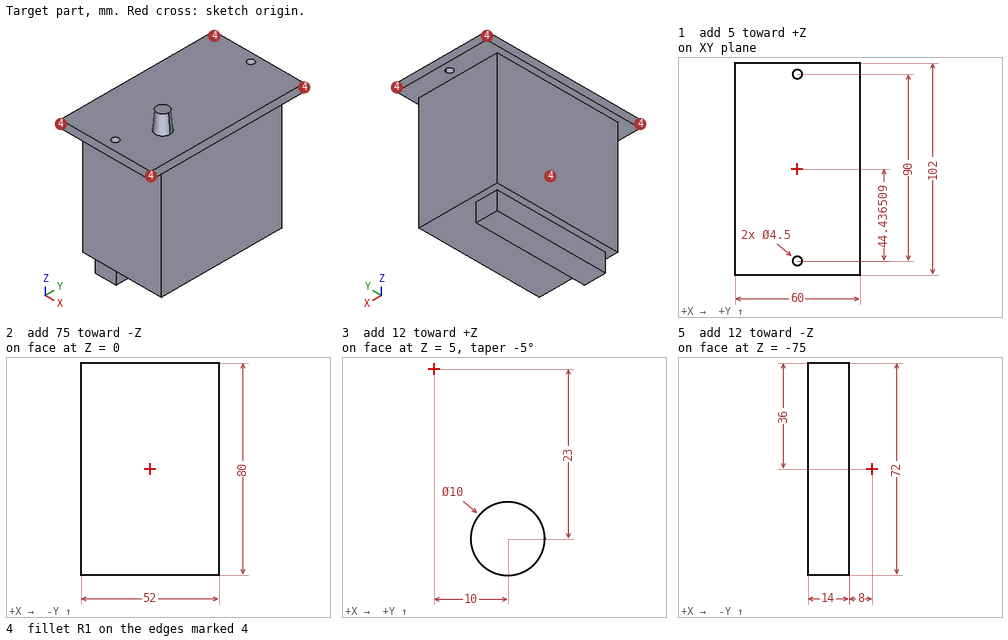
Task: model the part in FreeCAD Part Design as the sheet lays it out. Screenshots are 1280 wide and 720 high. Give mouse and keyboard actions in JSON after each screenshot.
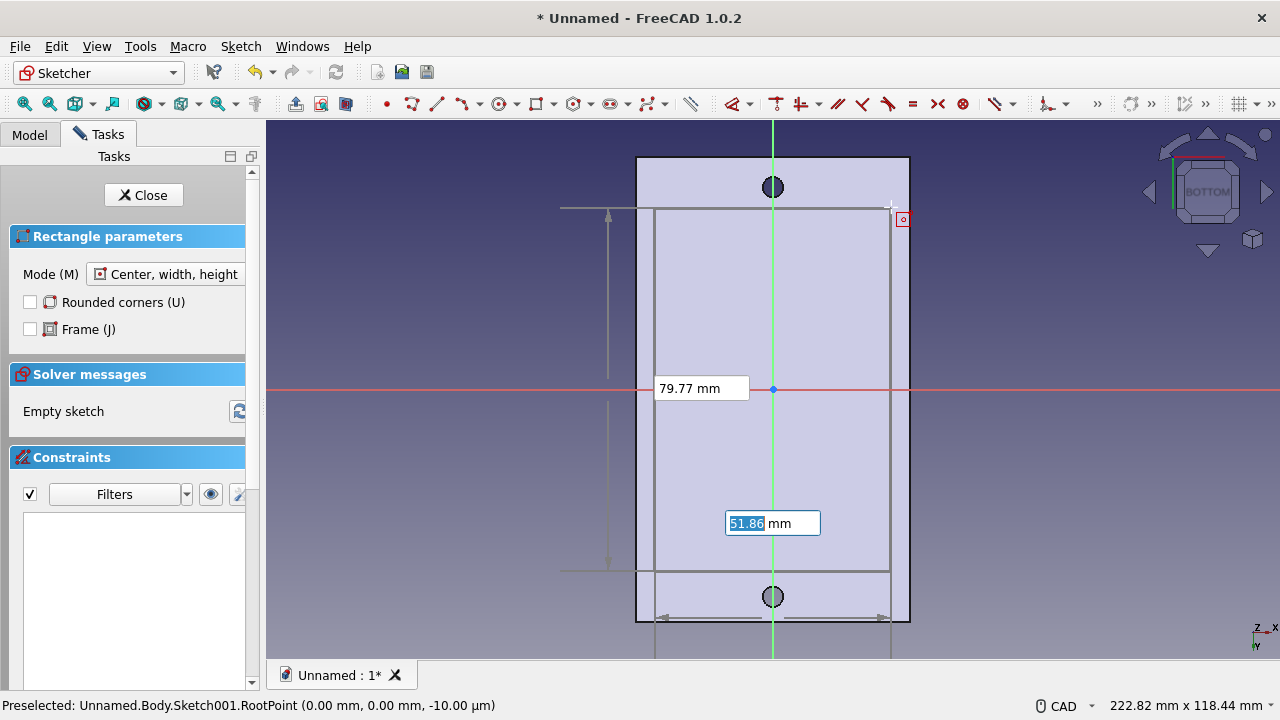
{"action": "type", "text": "52"}
{"action": "key", "text": "Tab"}
{"action": "type", "text": "80"}
{"action": "key", "text": "Return"}
{"action": "key", "text": "Escape"}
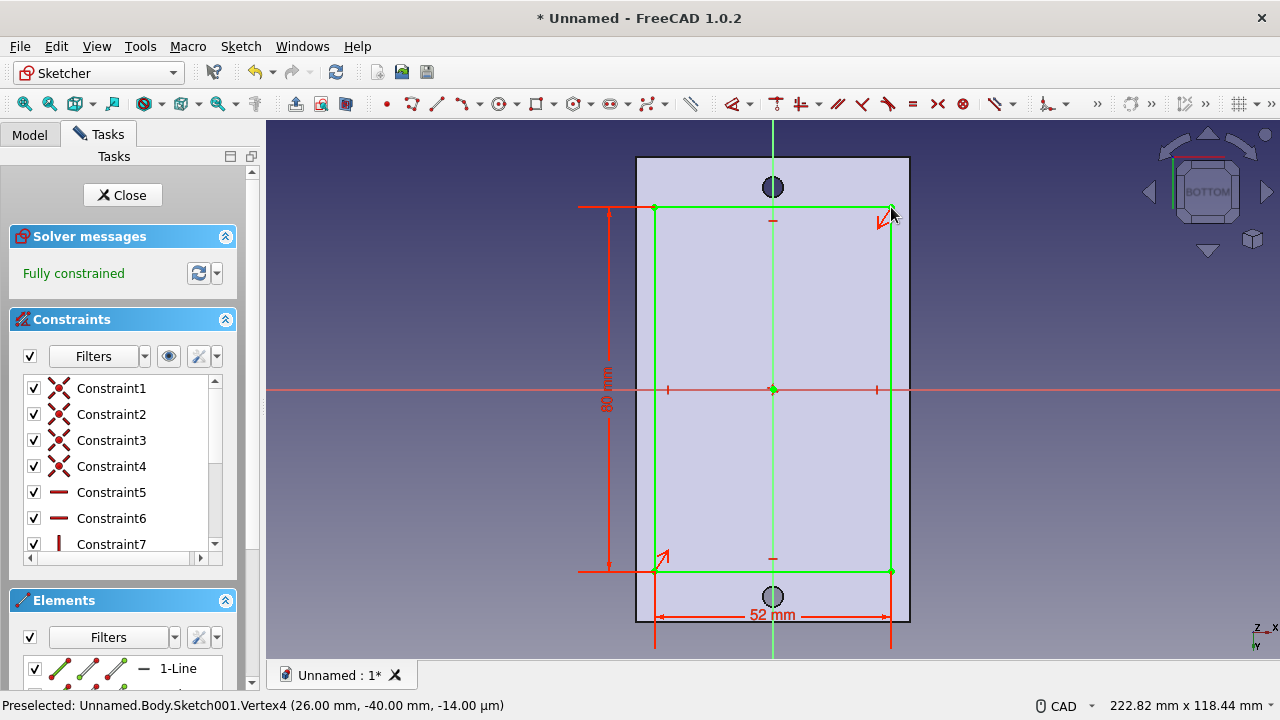
{"action": "left_click", "coordinate": [123, 195]}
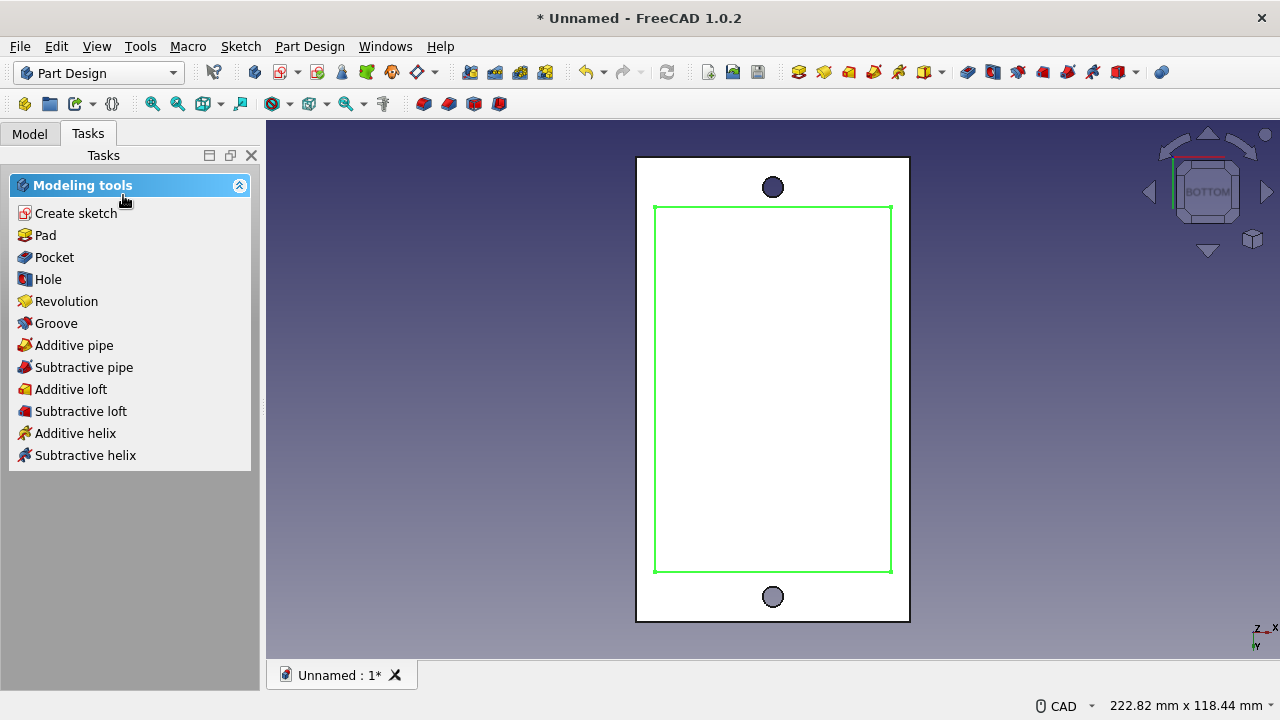
{"action": "left_click", "coordinate": [799, 72]}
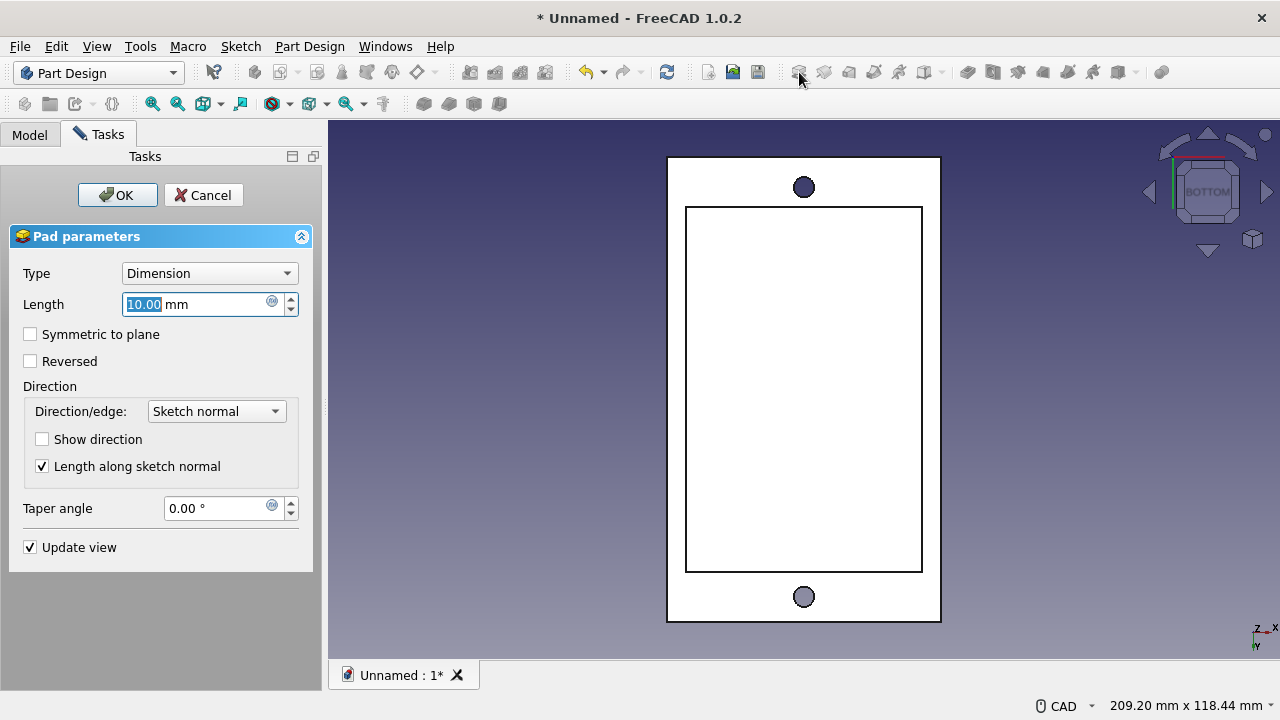
{"action": "type", "text": "75"}
{"action": "key", "text": "Tab"}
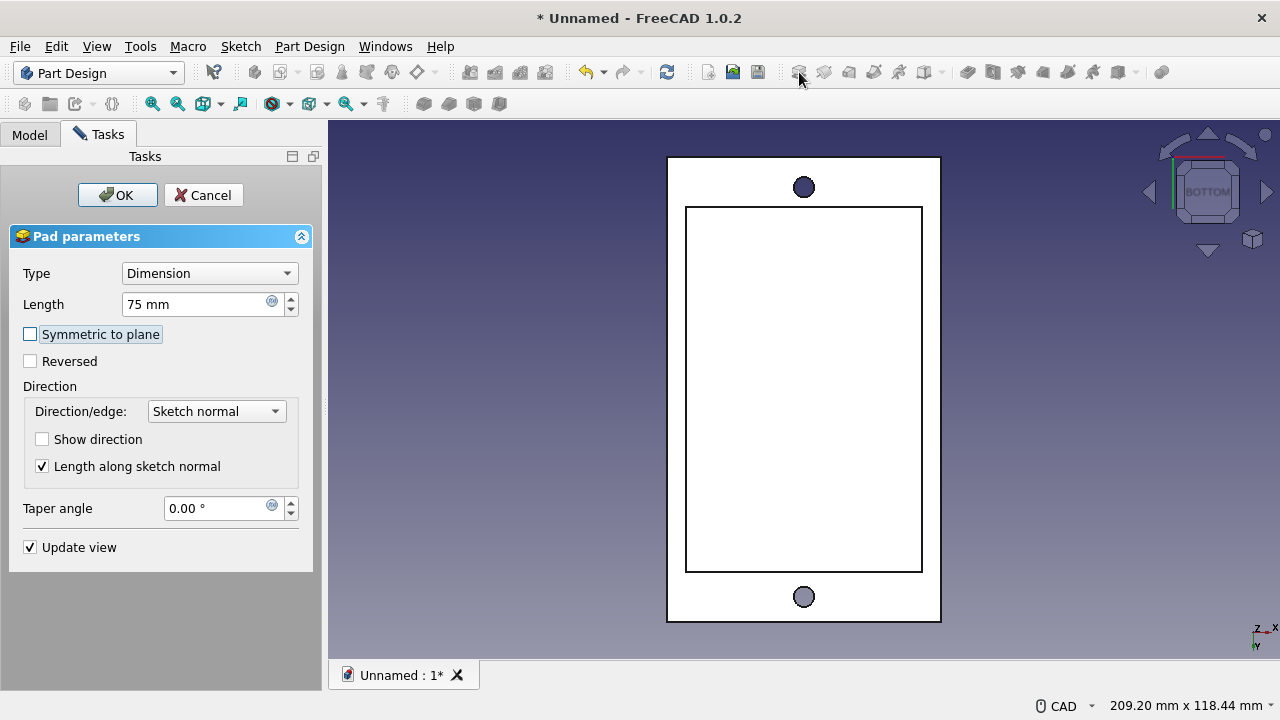
{"action": "left_click", "coordinate": [118, 195]}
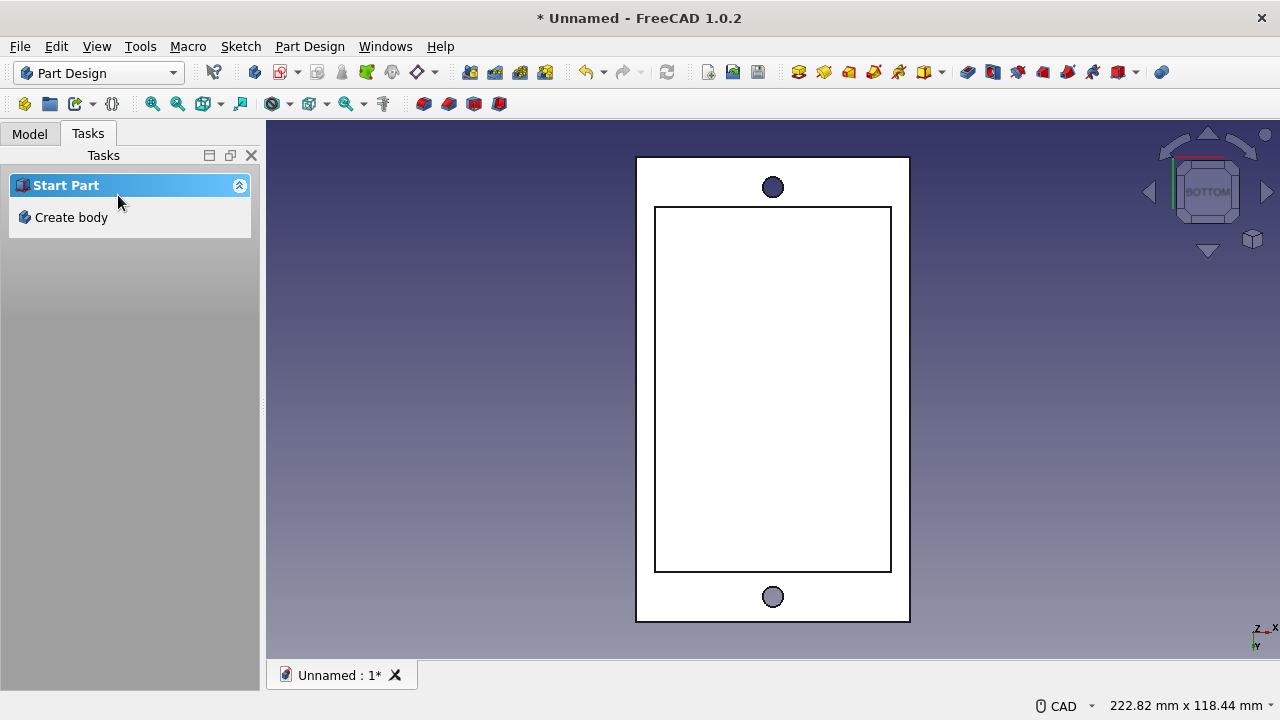
{"action": "key", "text": "0"}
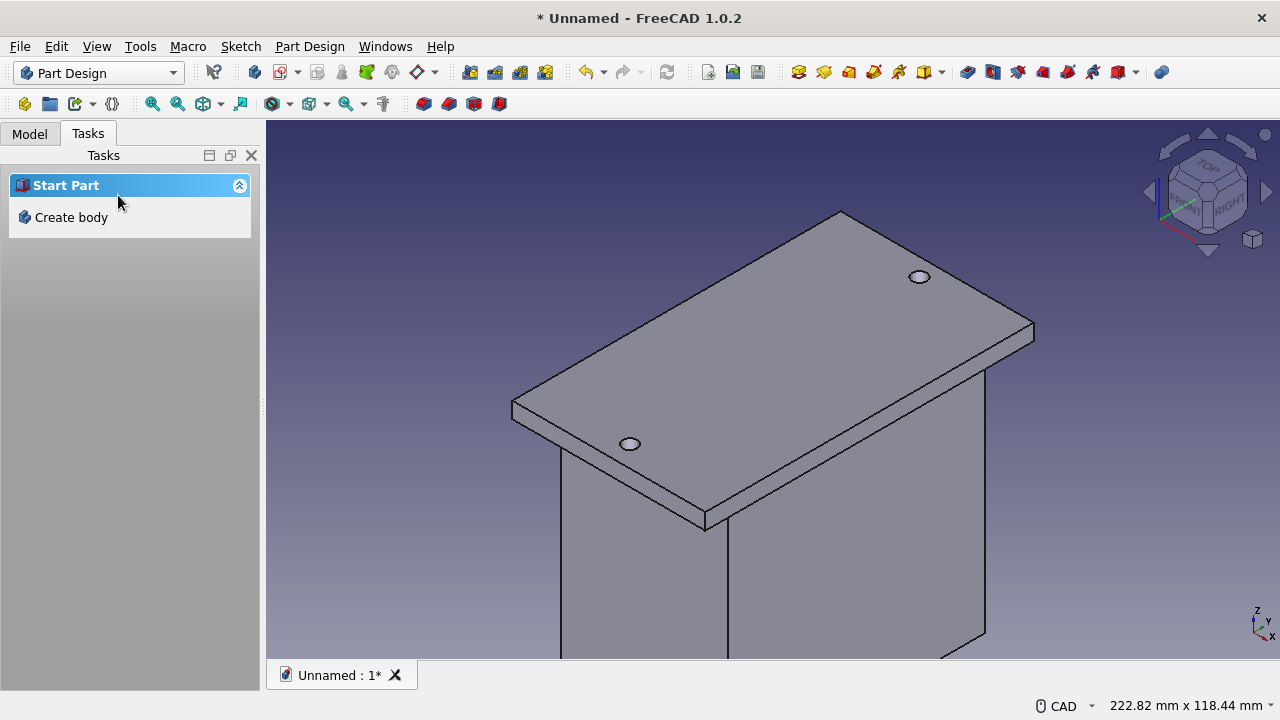
{"action": "key", "text": "v f"}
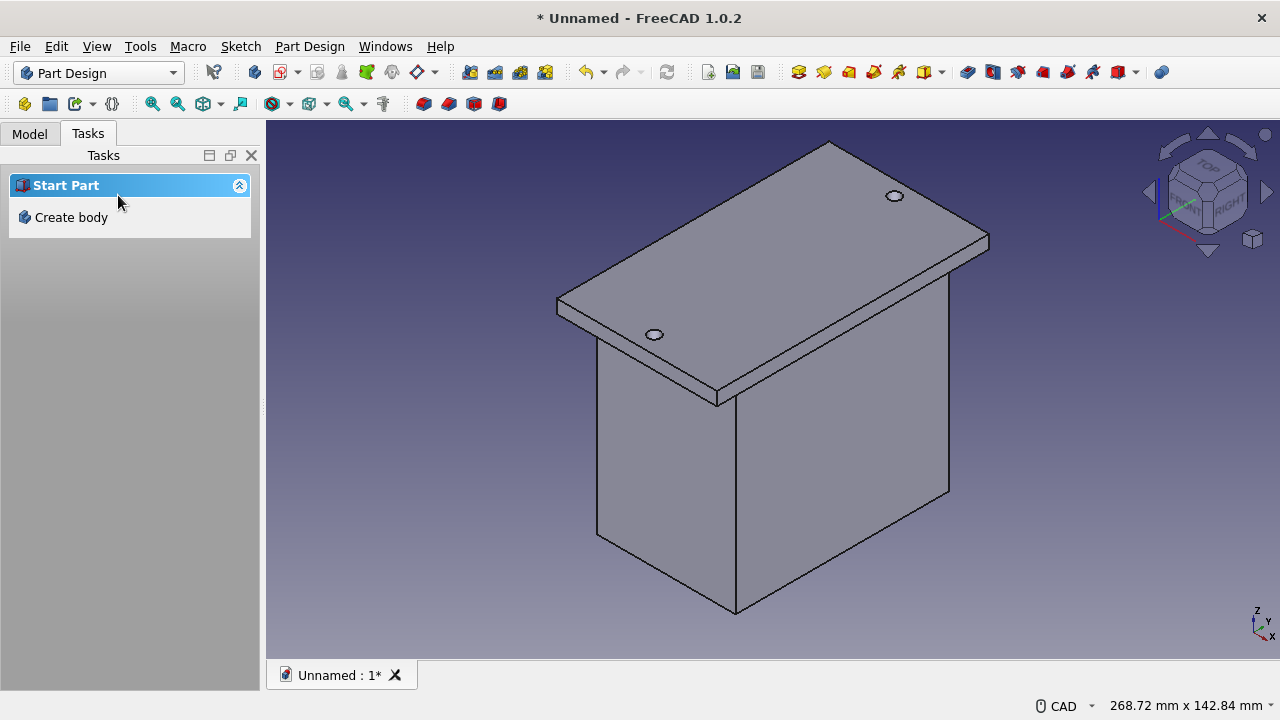
{"action": "left_click", "coordinate": [773, 265]}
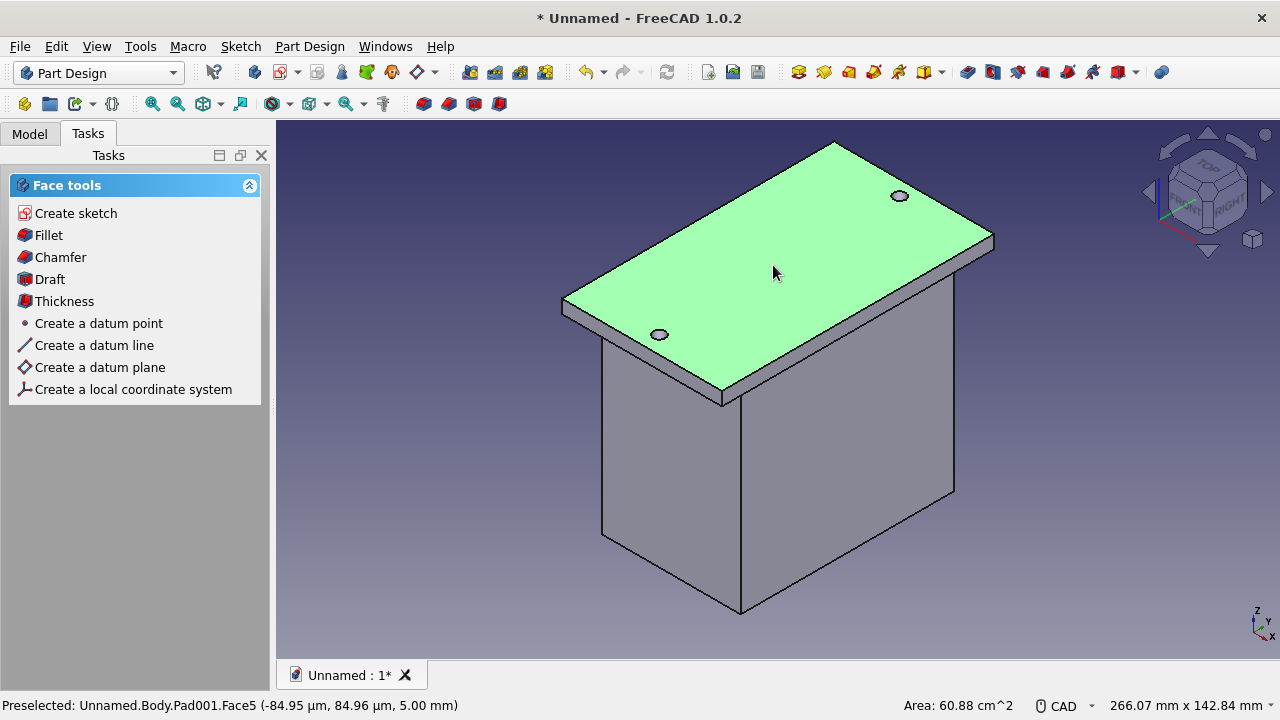
{"action": "left_click", "coordinate": [280, 72]}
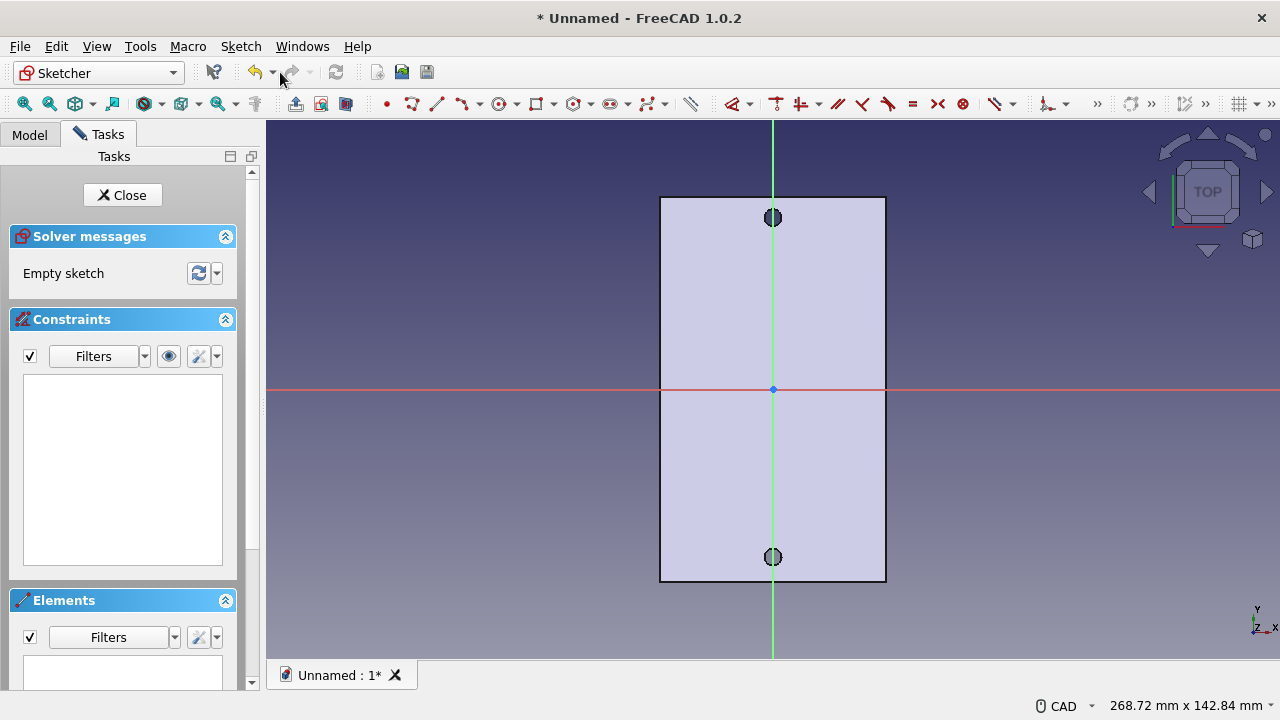
{"action": "scroll", "coordinate": [824, 487], "scroll_direction": "up", "scroll_amount": 11}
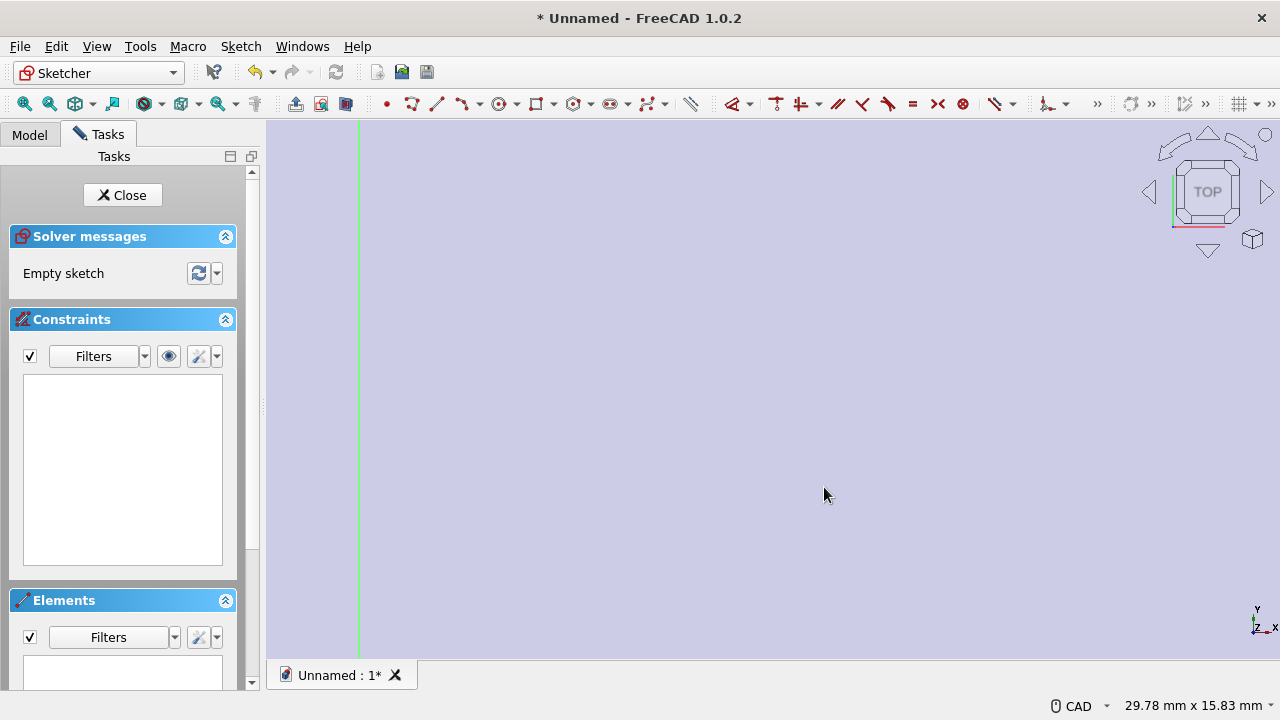
{"action": "key", "text": "g c"}